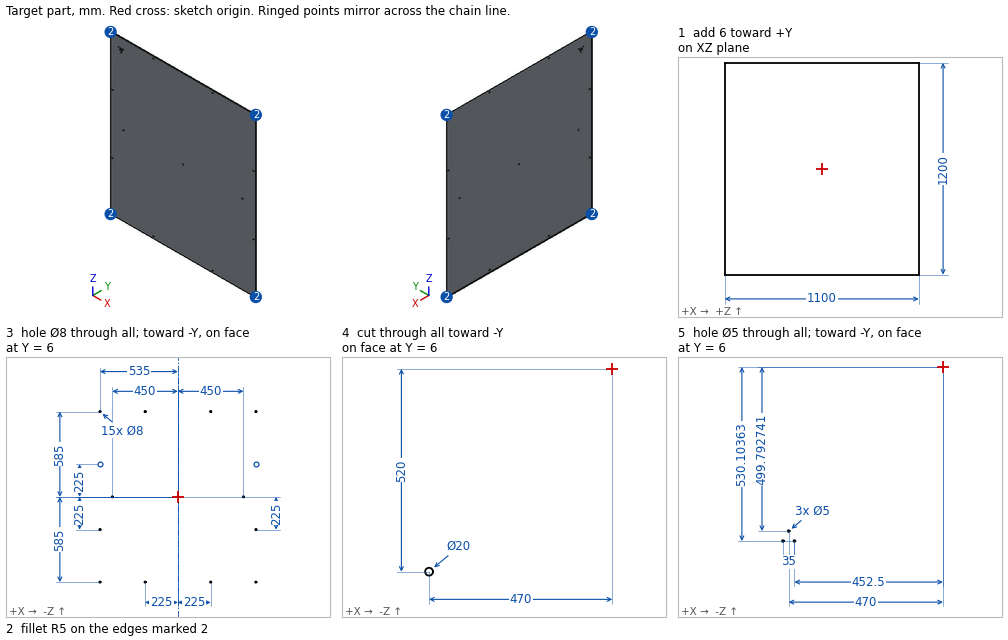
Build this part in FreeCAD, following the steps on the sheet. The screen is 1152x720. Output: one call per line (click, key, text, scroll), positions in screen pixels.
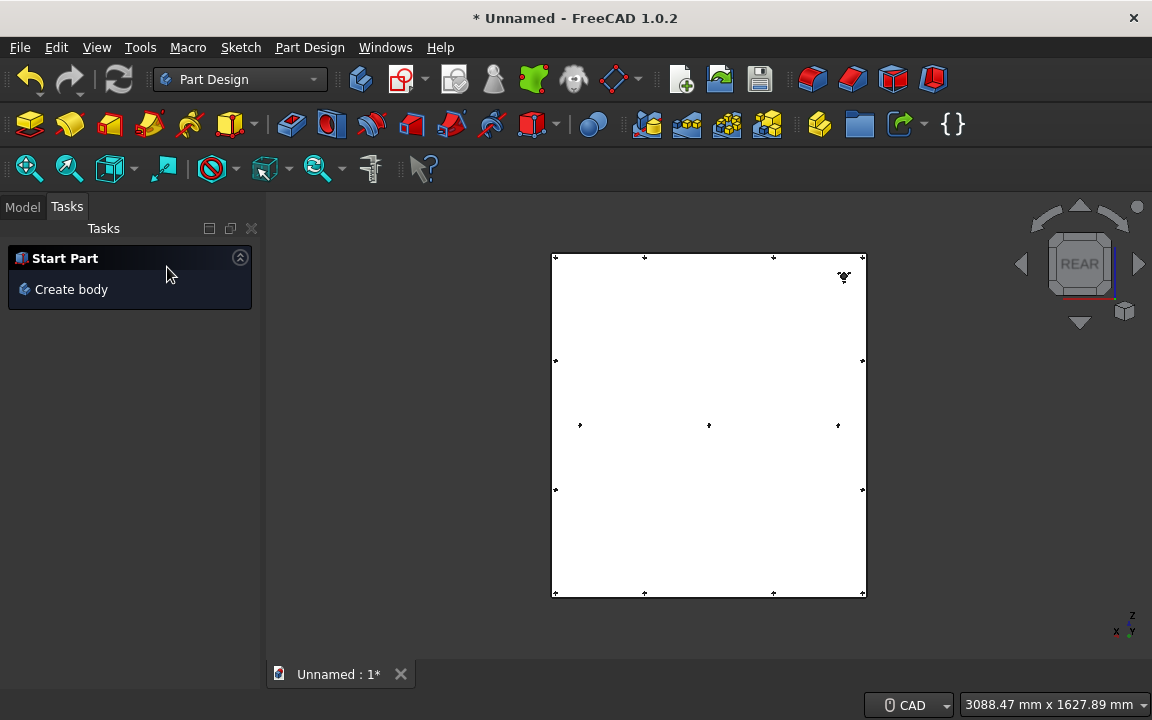
key(0)